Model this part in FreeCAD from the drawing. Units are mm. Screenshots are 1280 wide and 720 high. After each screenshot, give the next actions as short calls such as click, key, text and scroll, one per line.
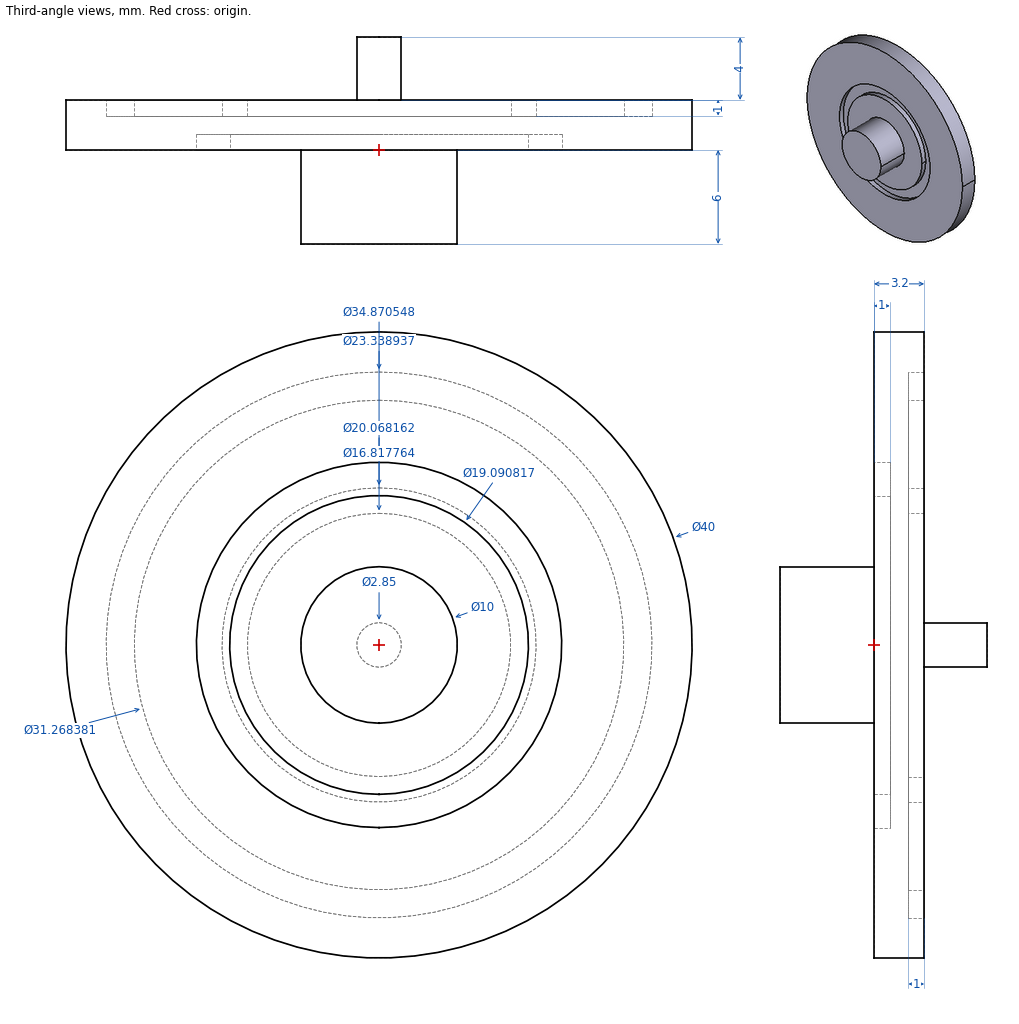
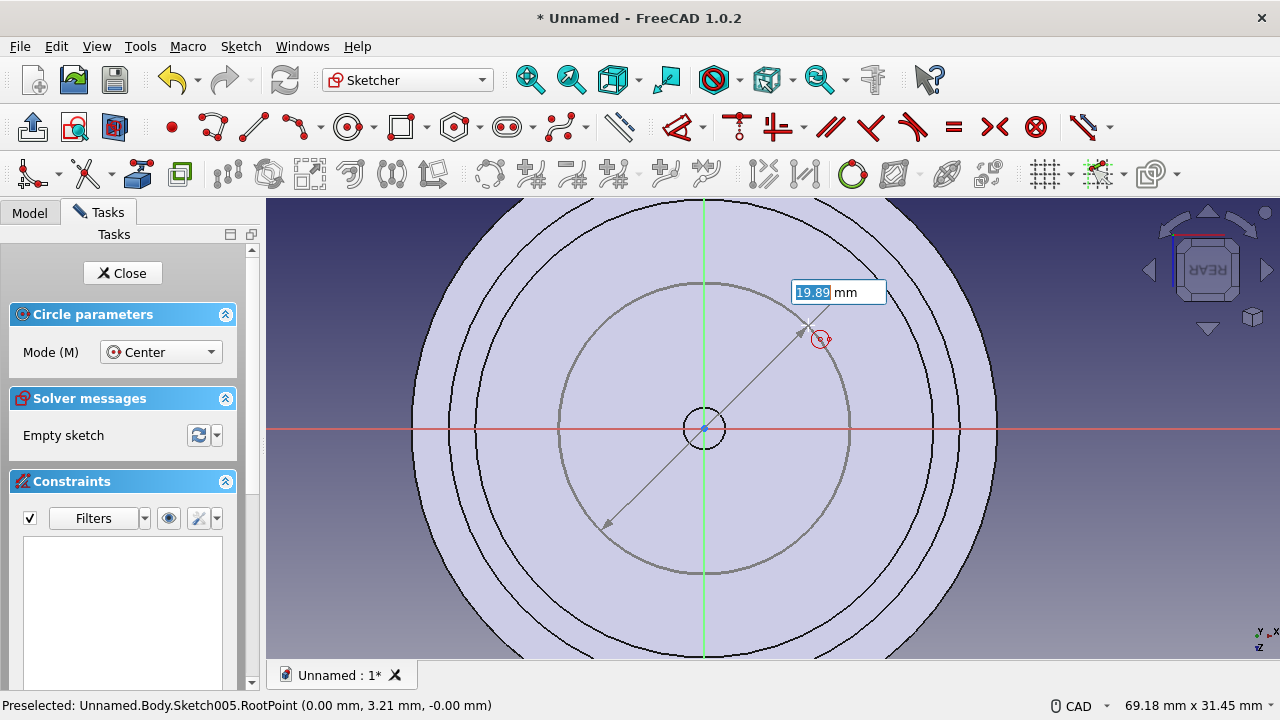
text(20.068162)
key(Return)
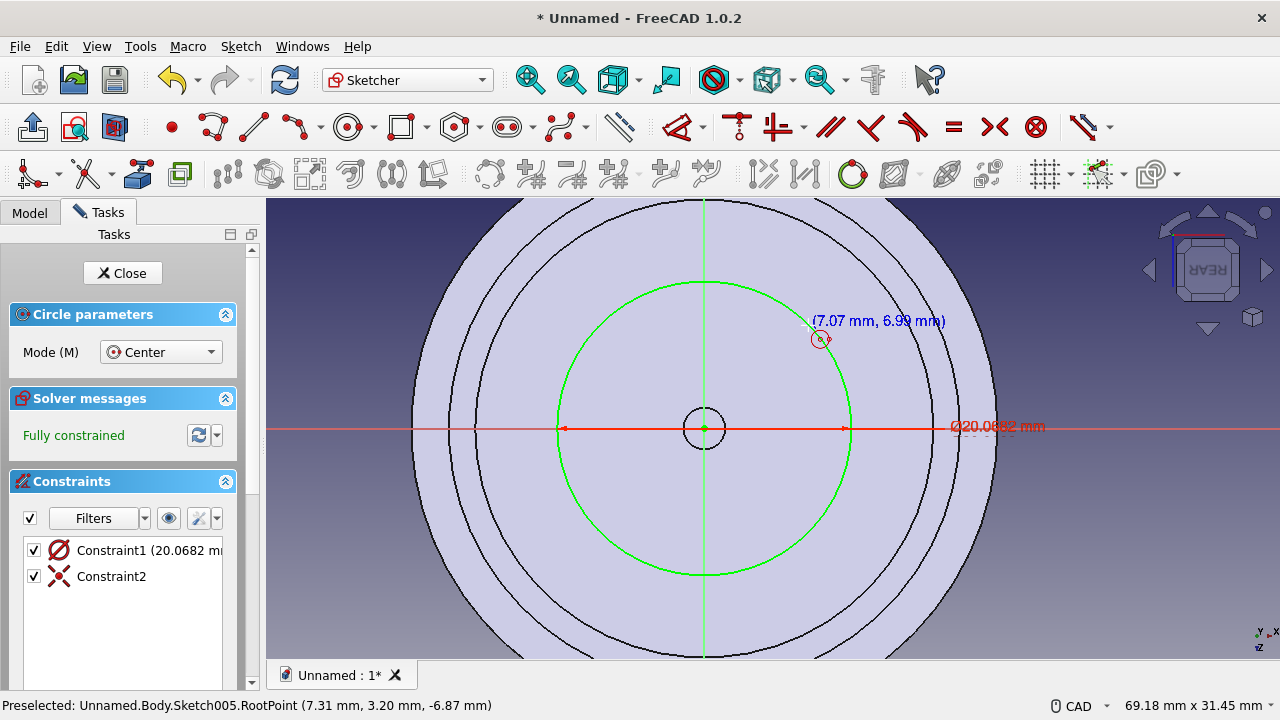
click(704, 428)
move(791, 341)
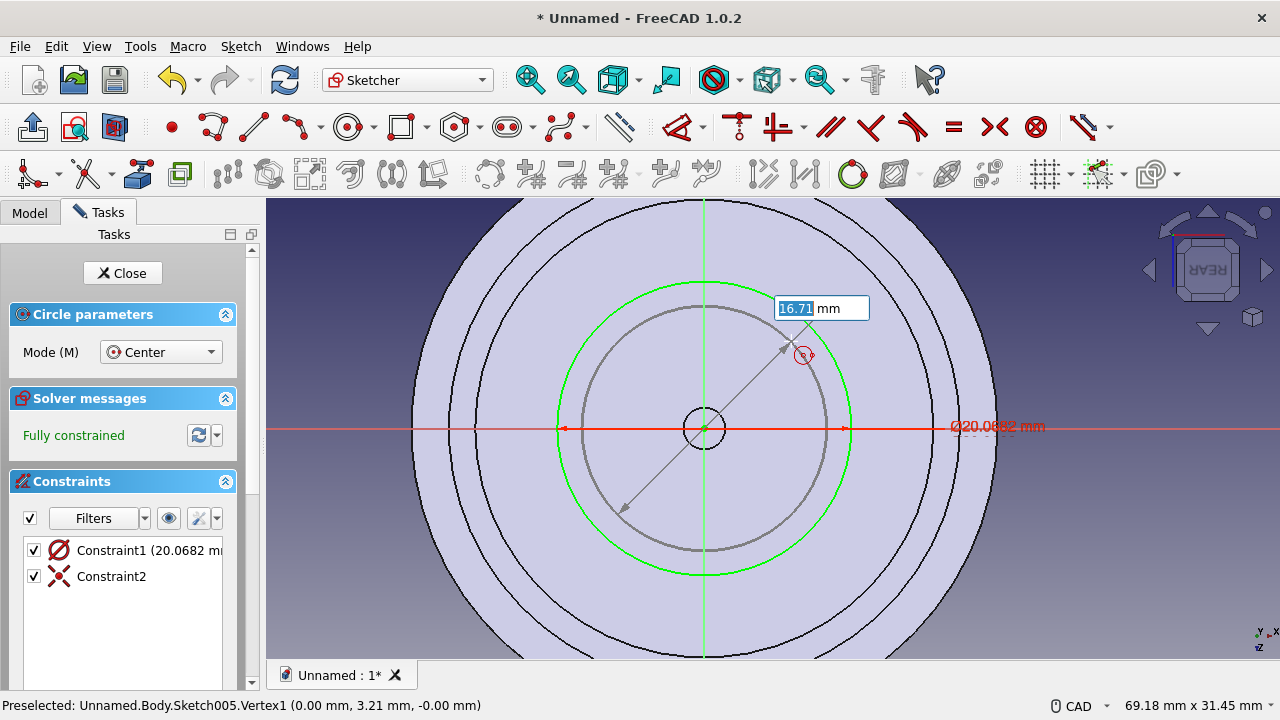
text(16.817764)
key(Return)
key(Escape)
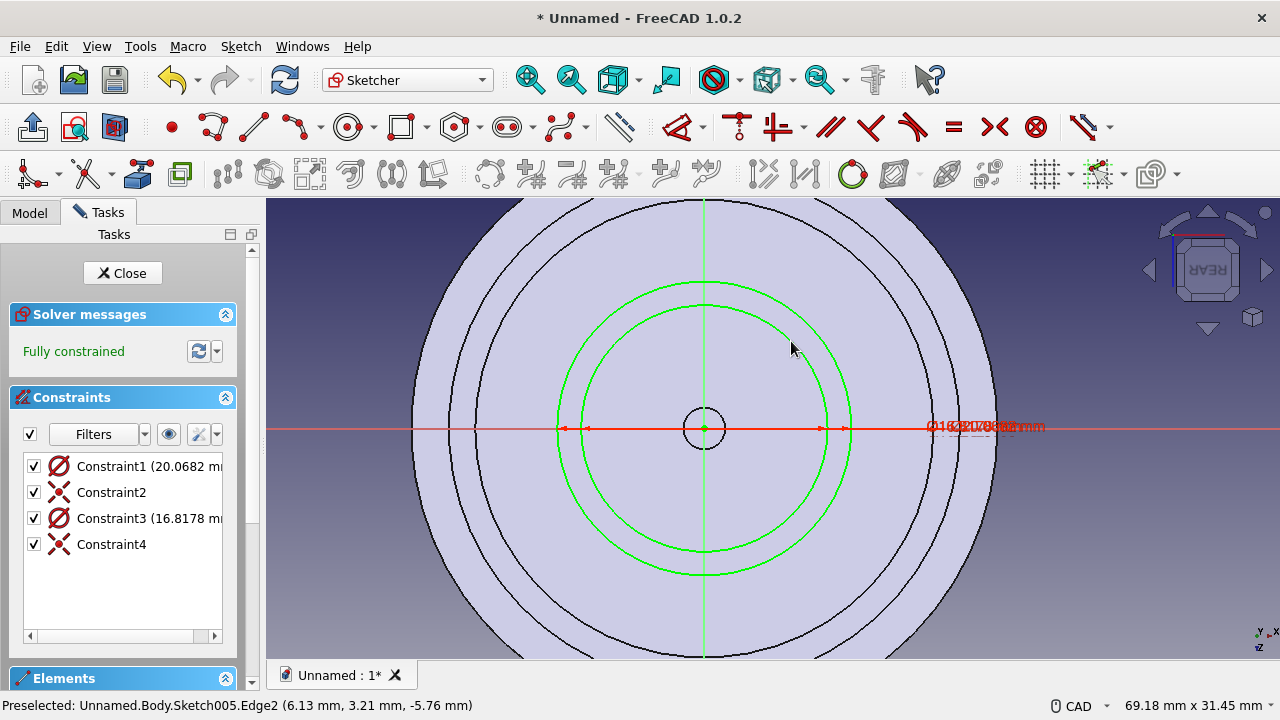
click(123, 273)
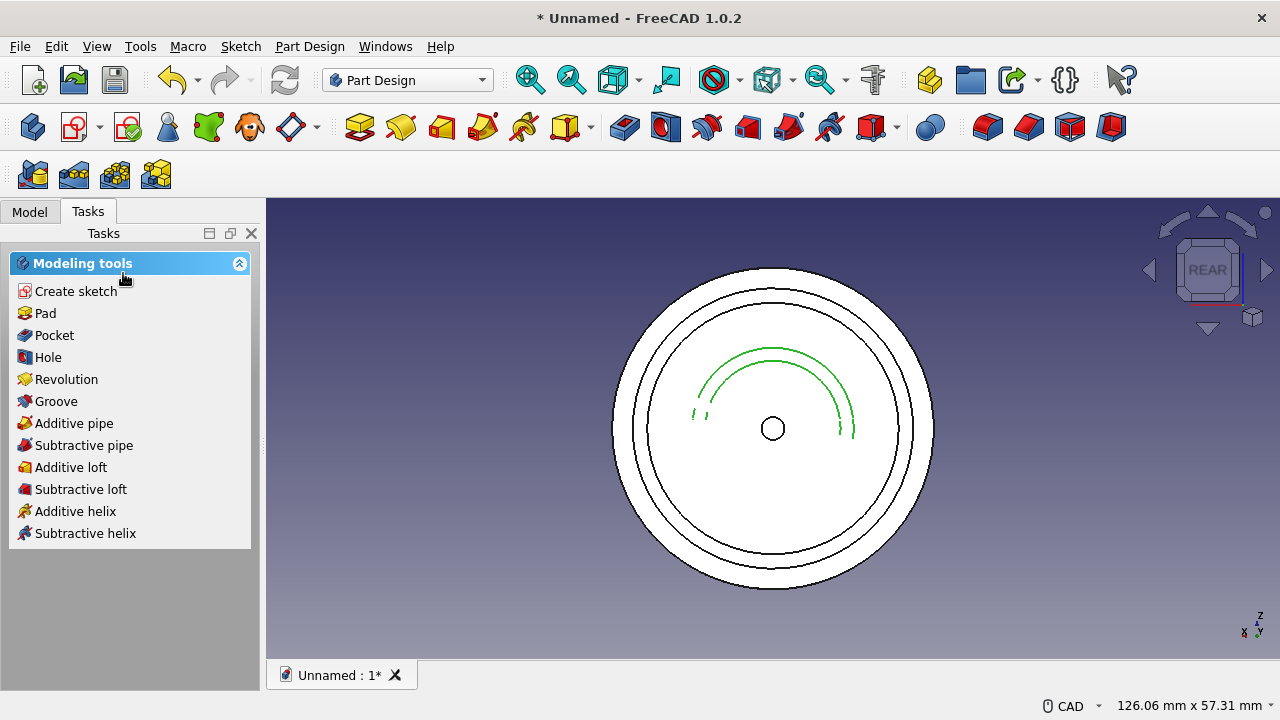
click(625, 128)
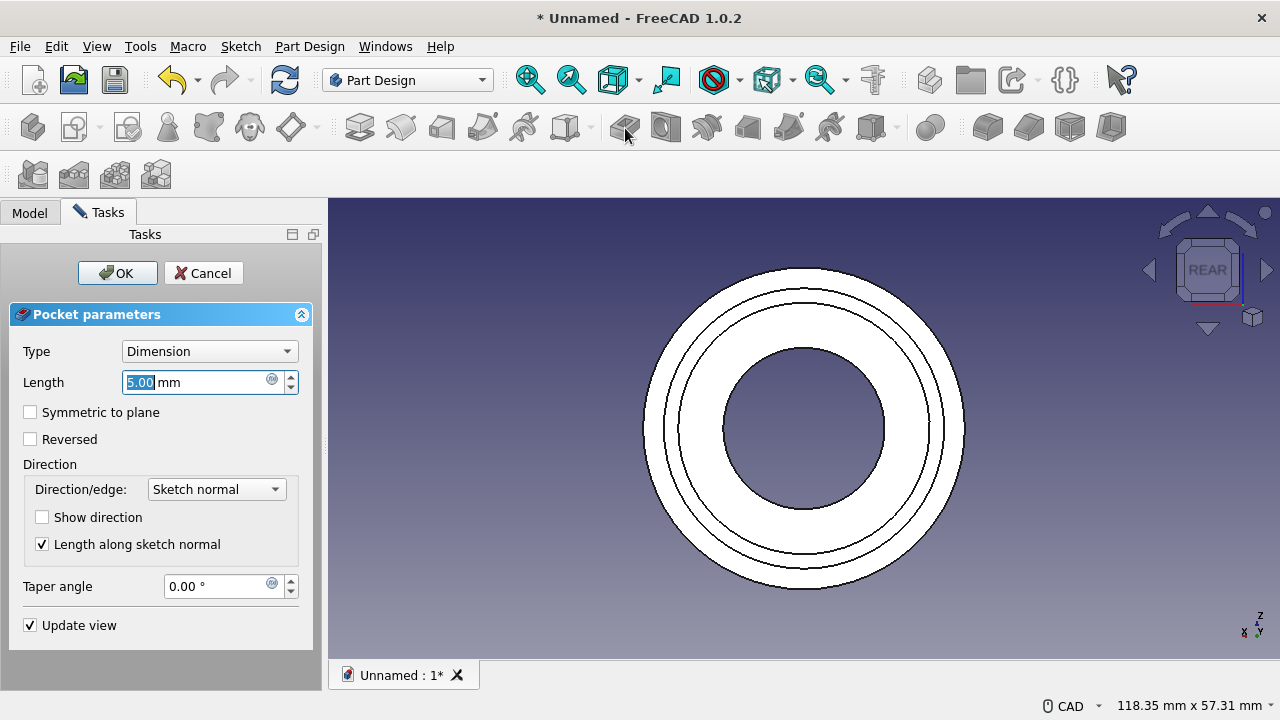
text(1)
key(Tab)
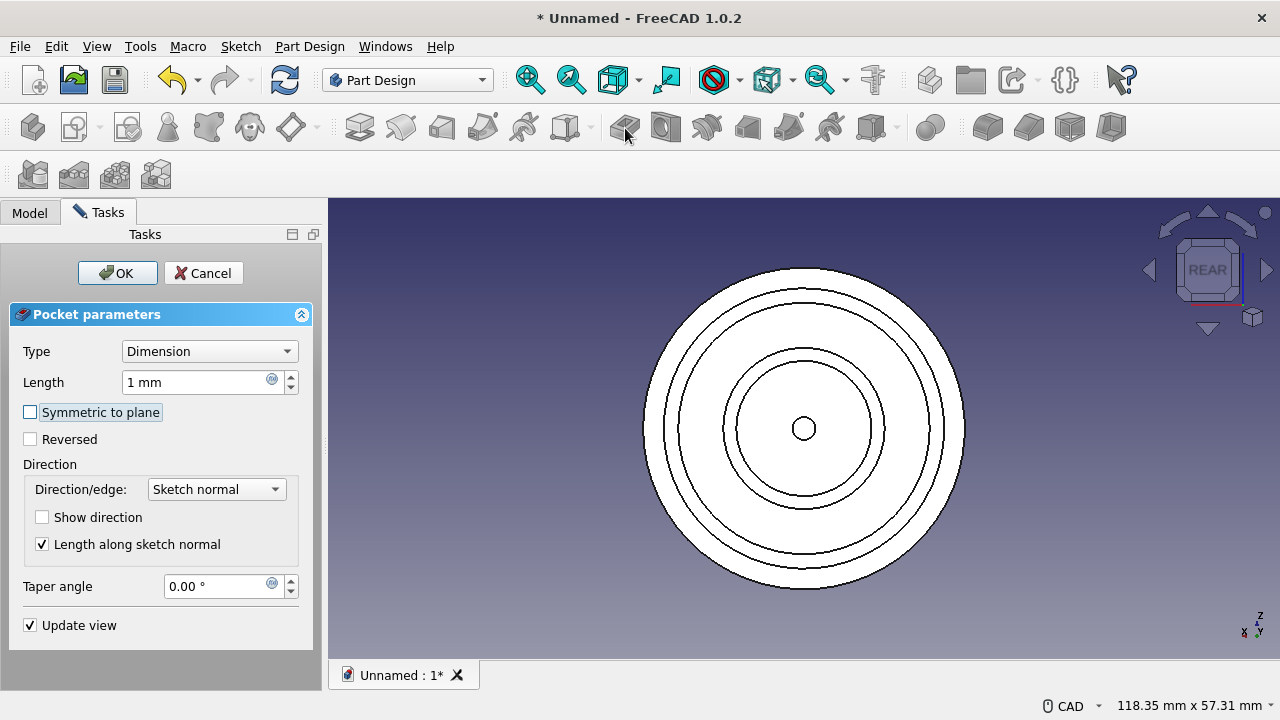
click(118, 273)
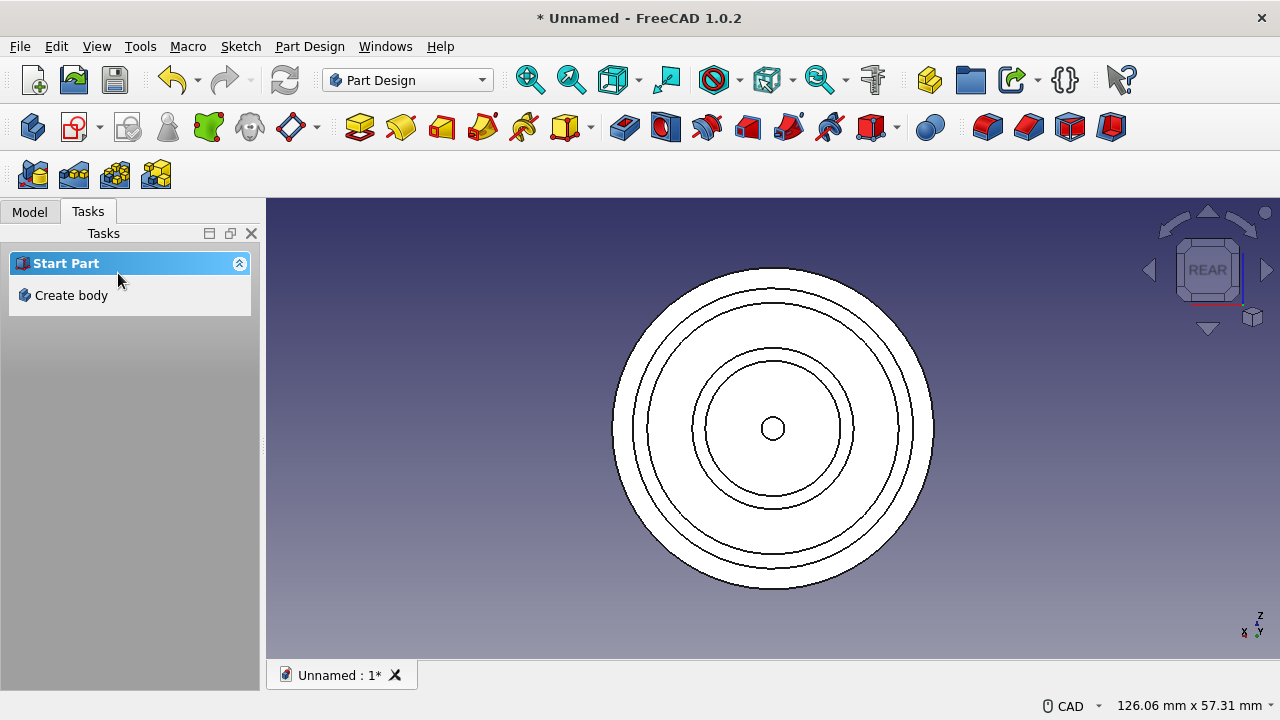
key(0)